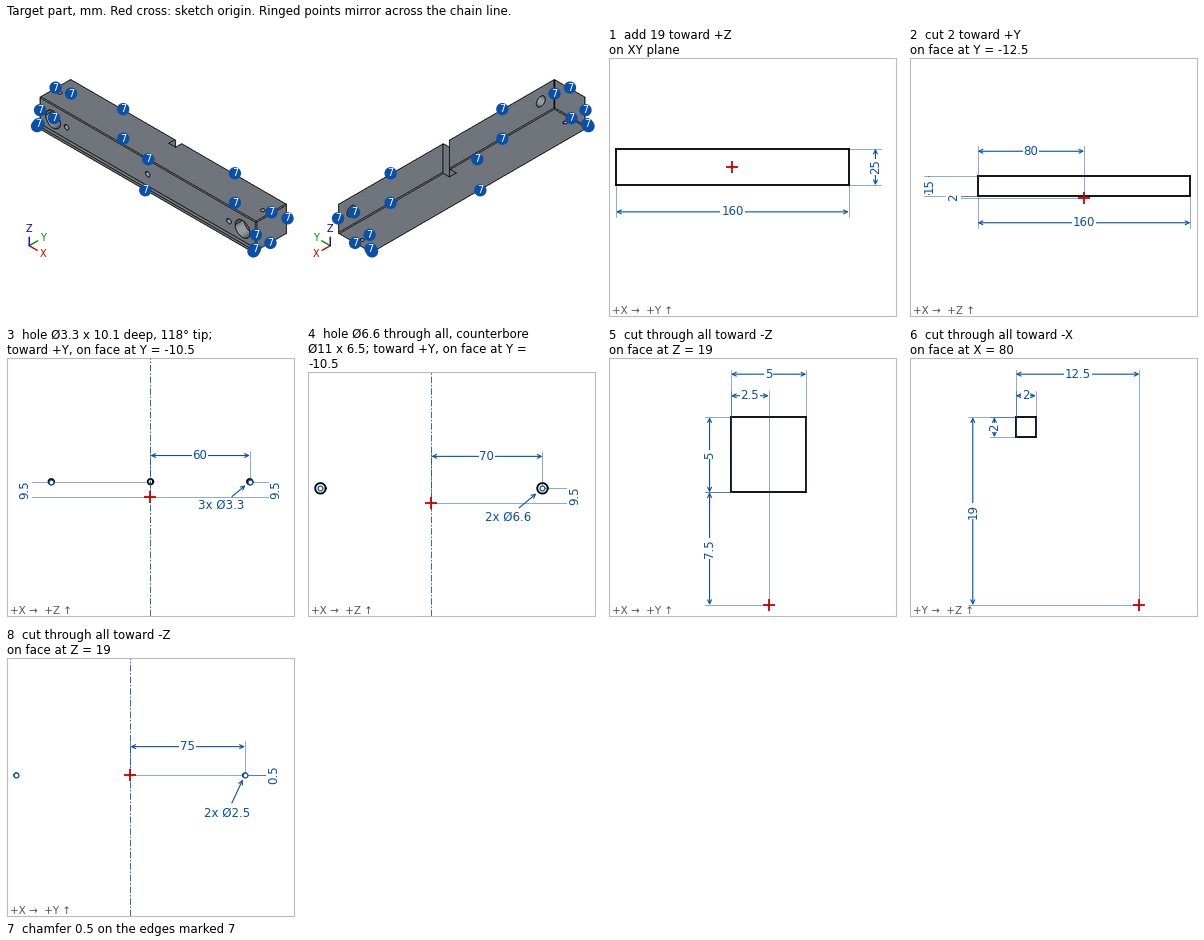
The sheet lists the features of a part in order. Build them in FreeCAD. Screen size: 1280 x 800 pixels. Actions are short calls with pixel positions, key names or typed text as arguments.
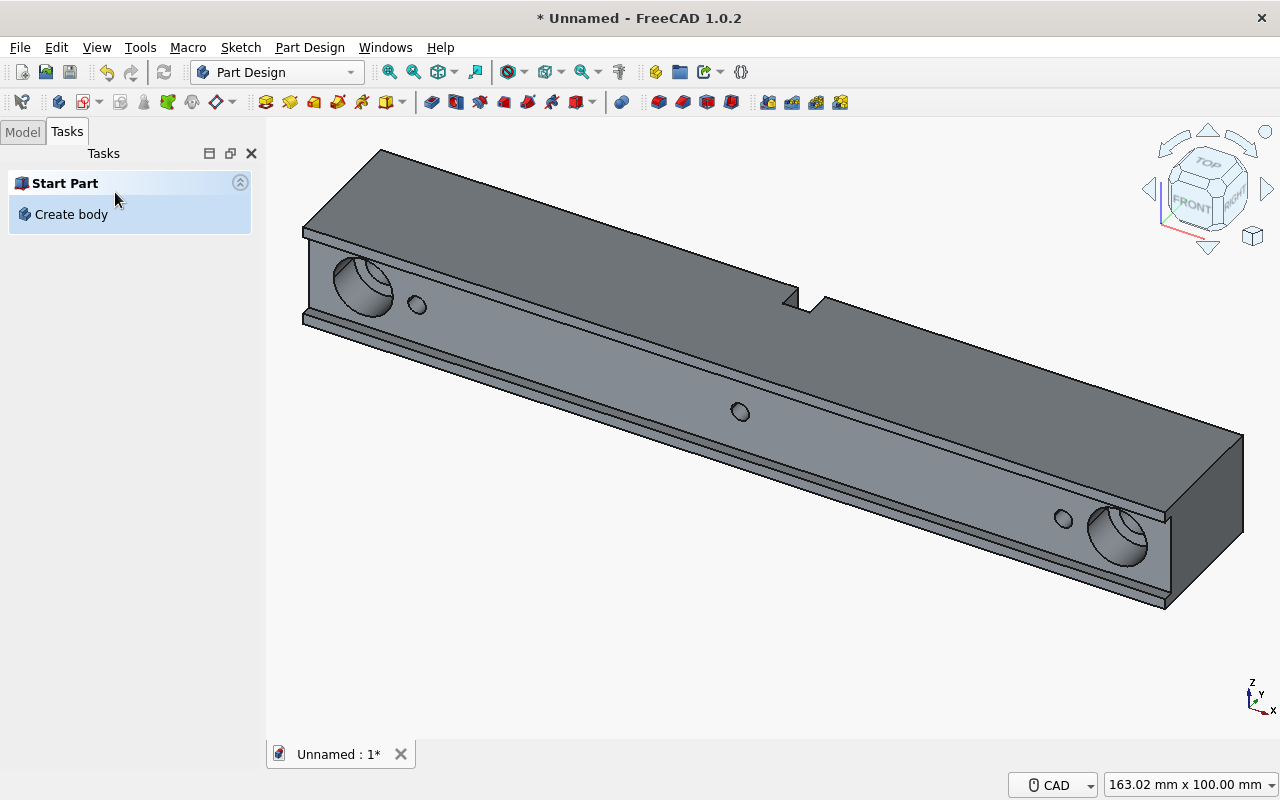
click(1204, 521)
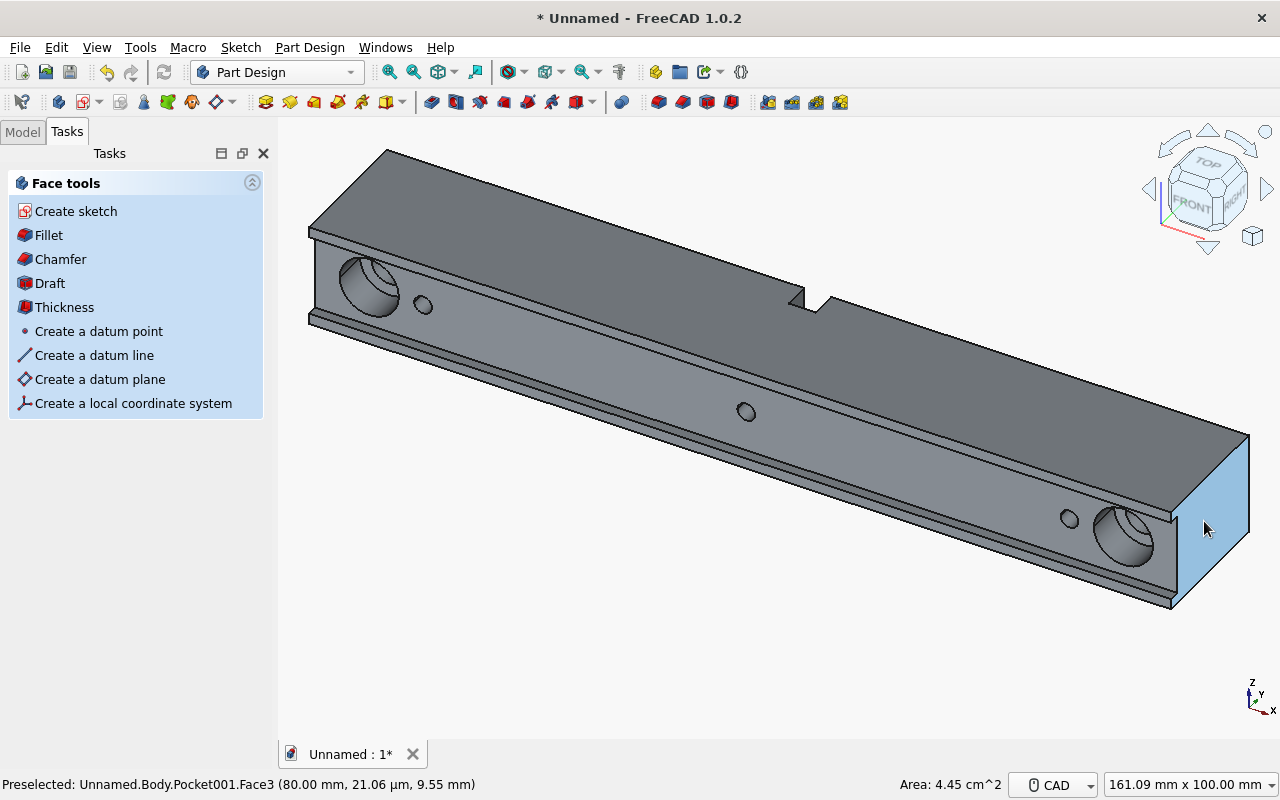
click(84, 102)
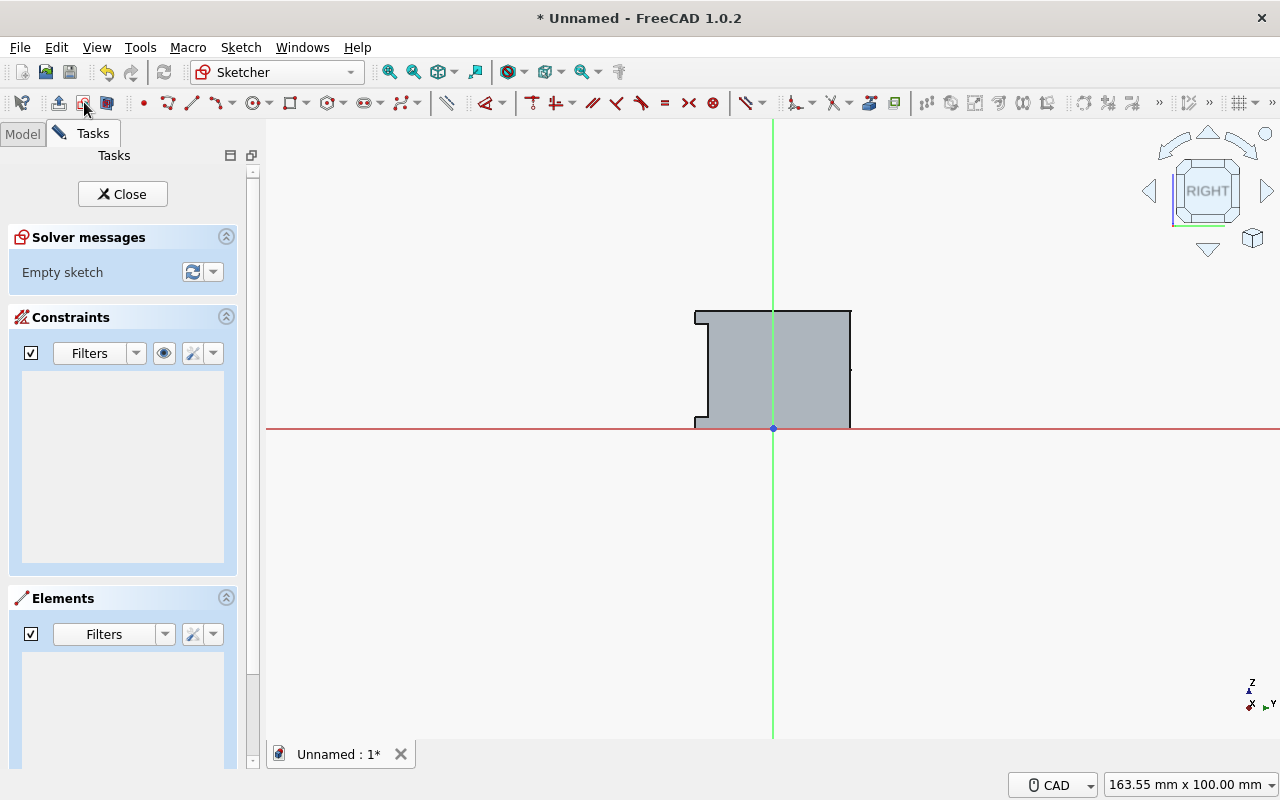
scroll(702, 312, up, 15)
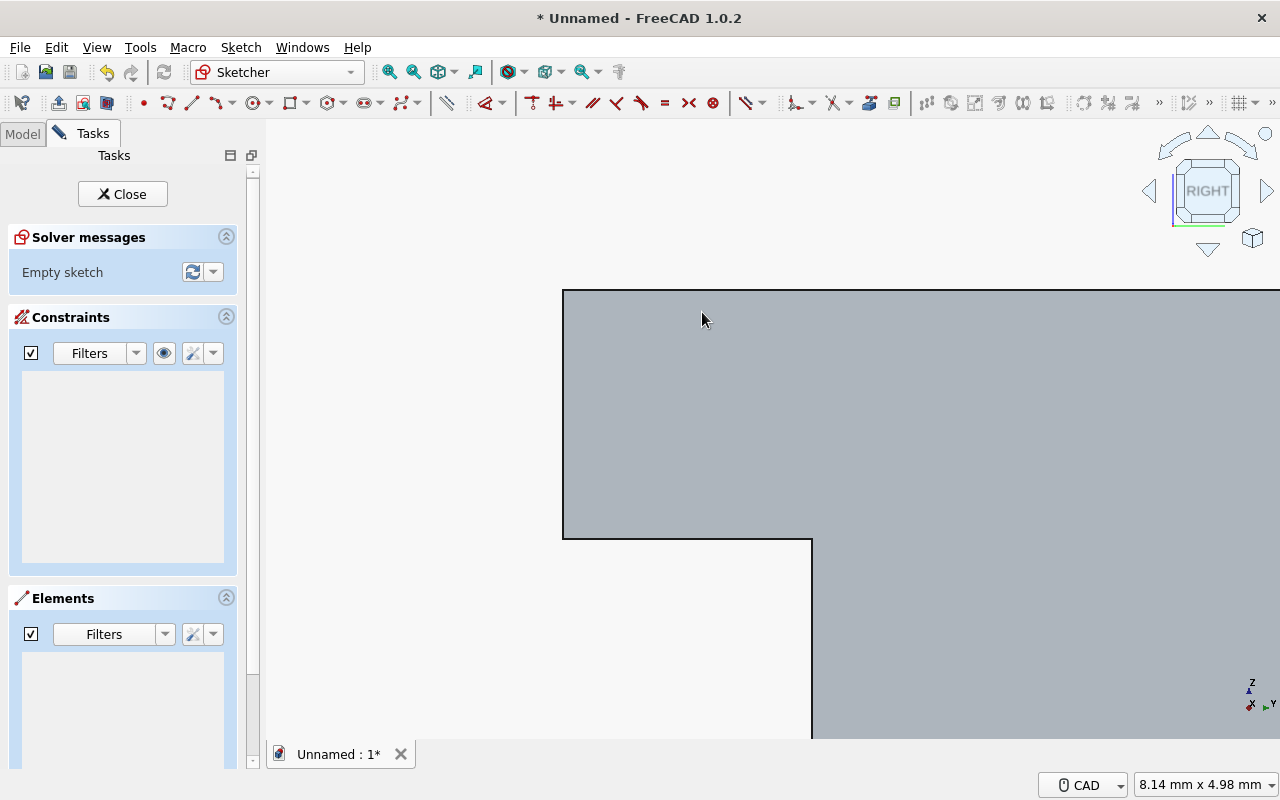
scroll(654, 385, up, 2)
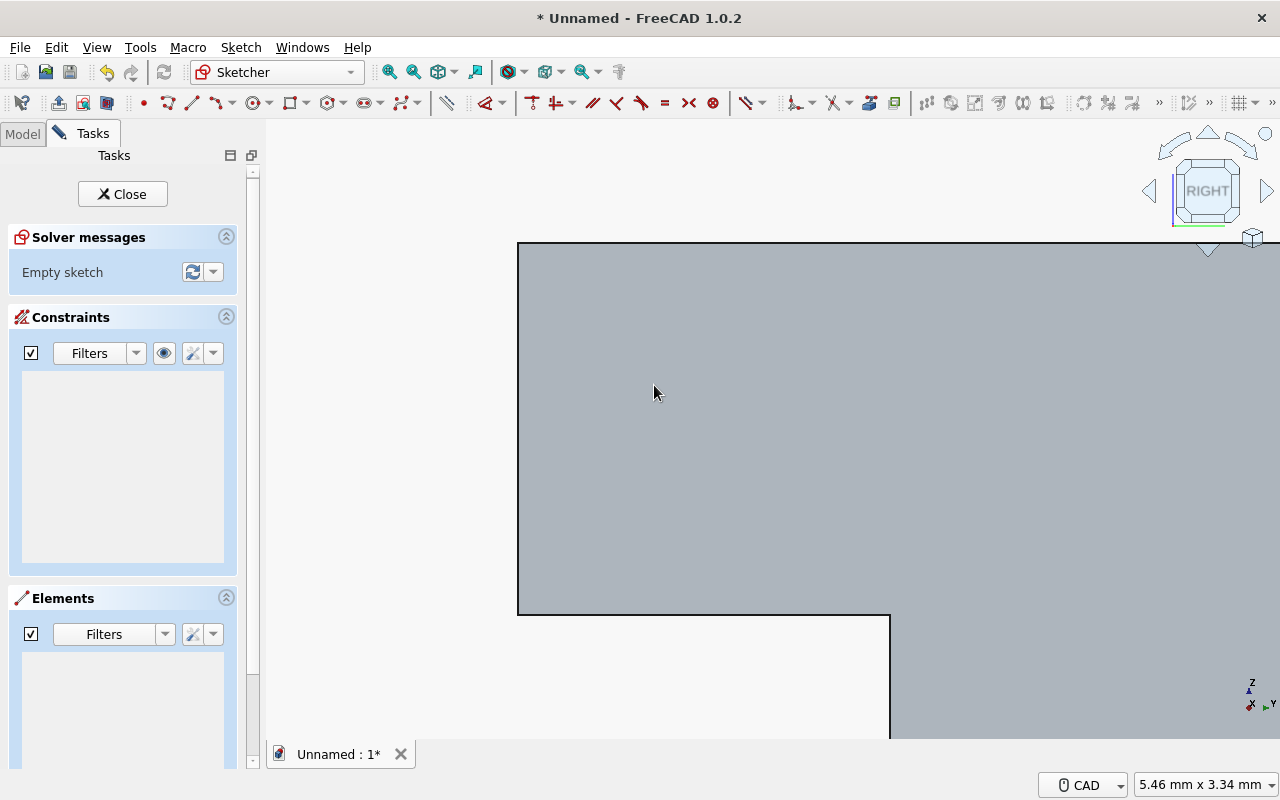
click(290, 104)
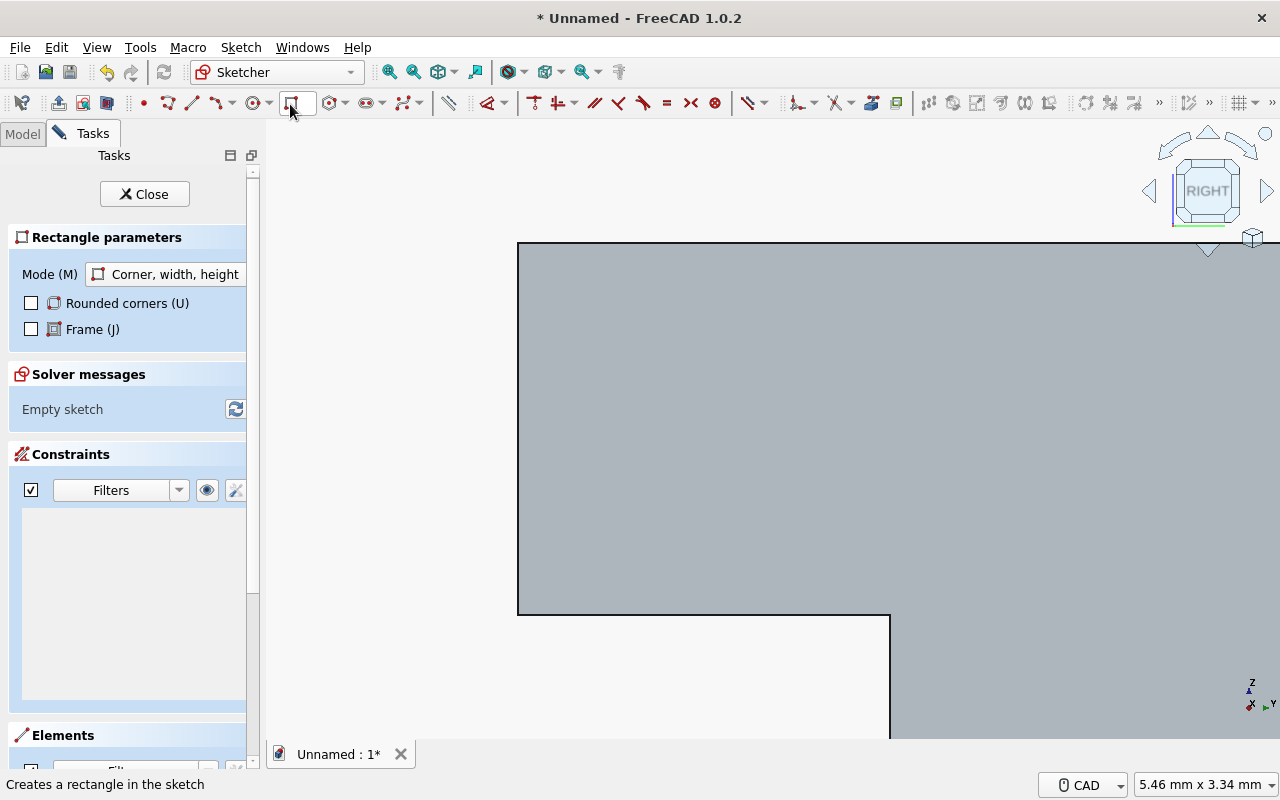
click(518, 243)
click(890, 615)
key(Escape)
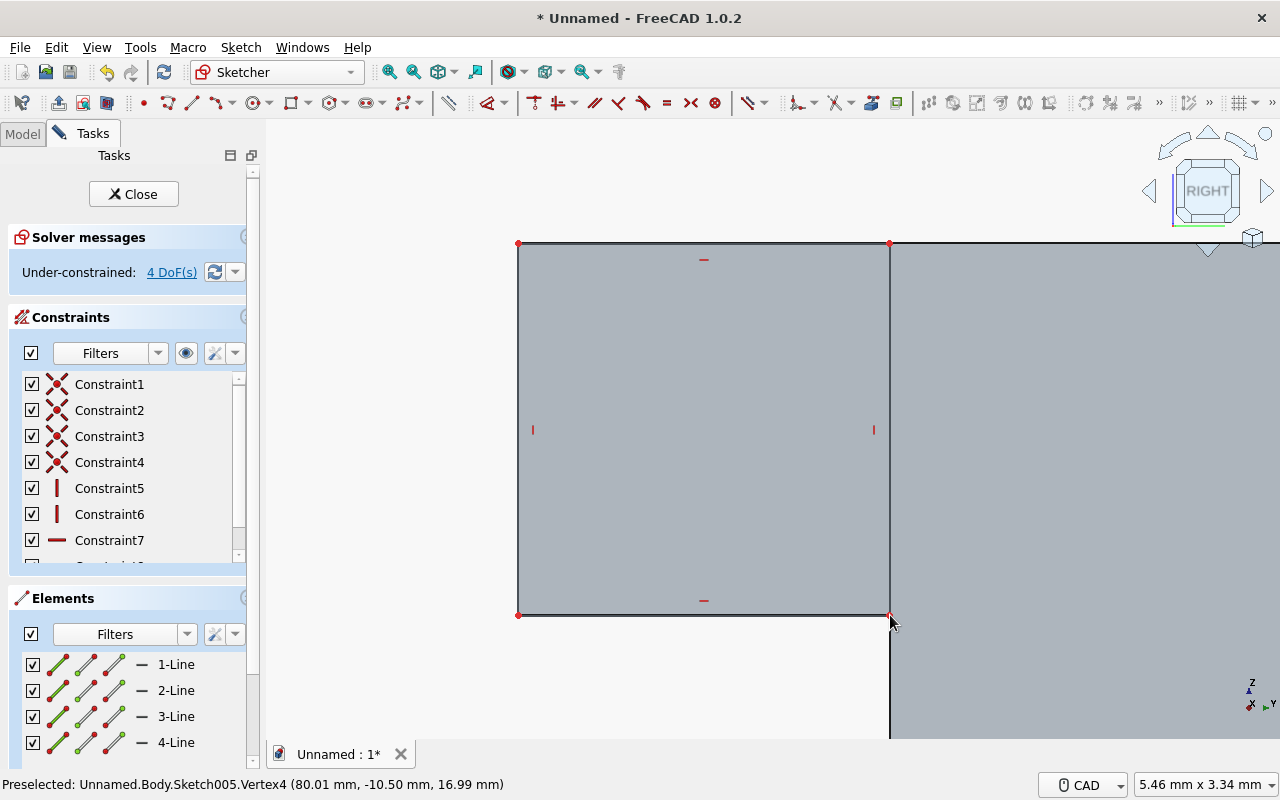
click(488, 104)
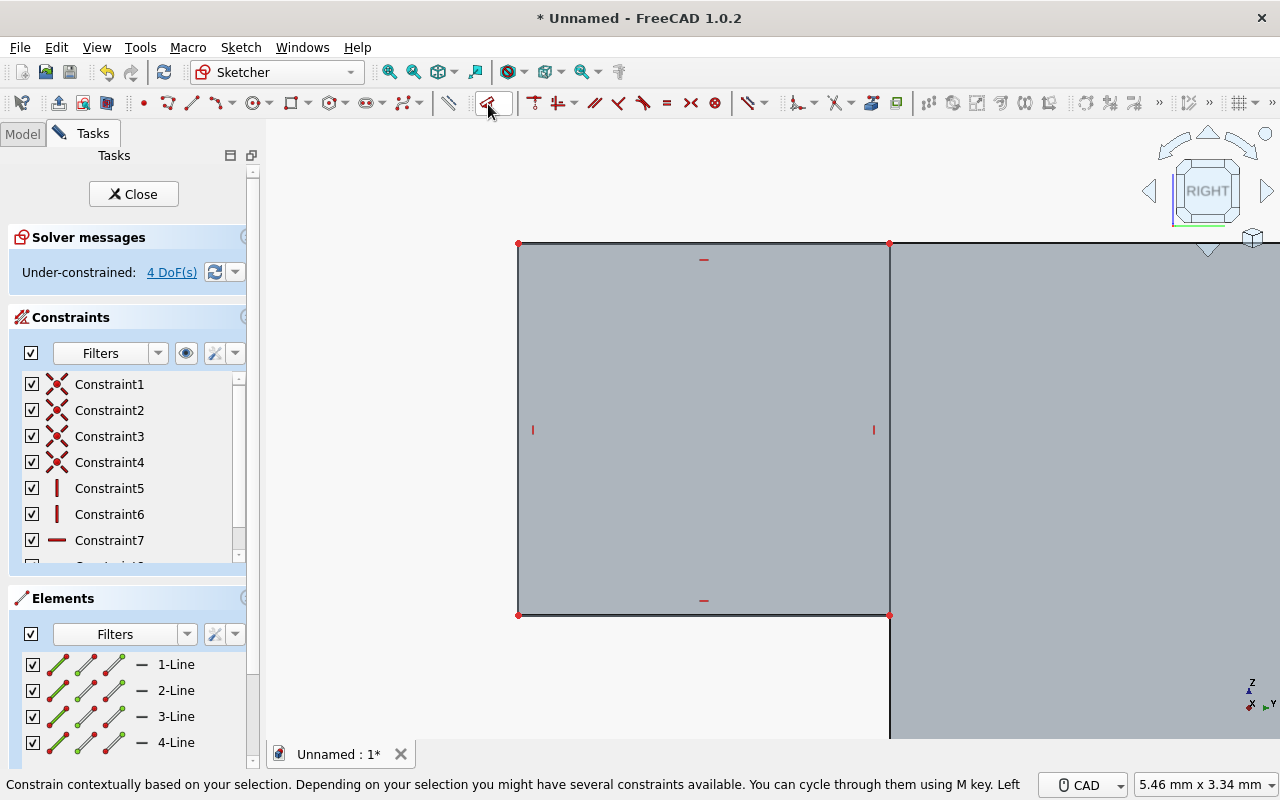
click(518, 356)
click(484, 430)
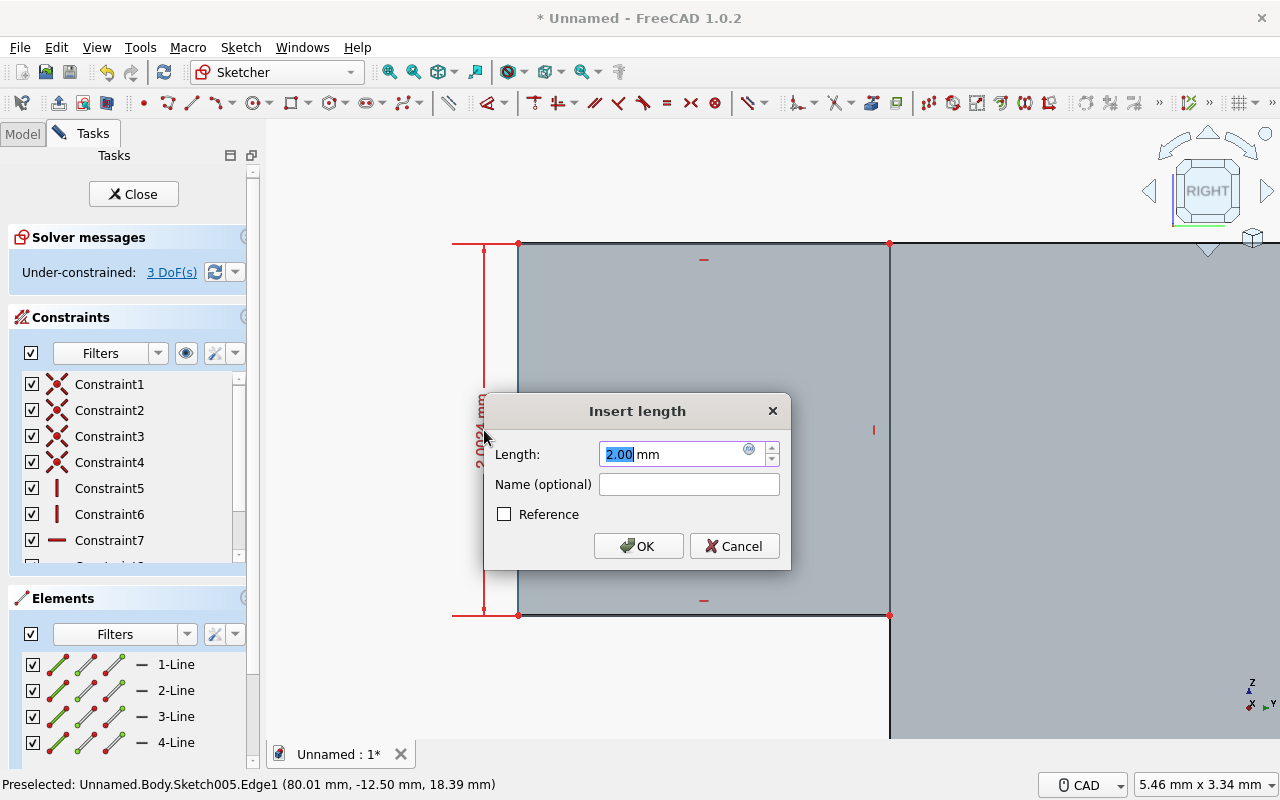
text(2)
key(Return)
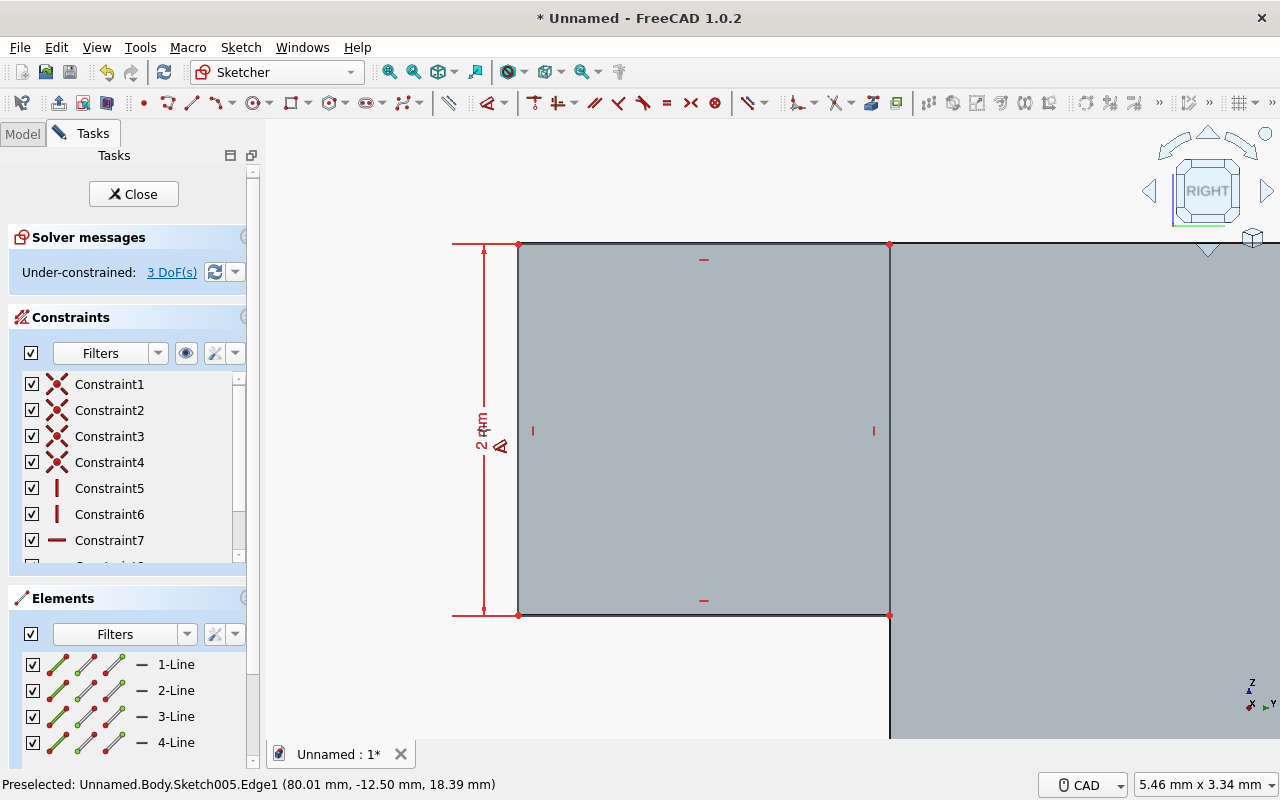
click(630, 616)
click(704, 650)